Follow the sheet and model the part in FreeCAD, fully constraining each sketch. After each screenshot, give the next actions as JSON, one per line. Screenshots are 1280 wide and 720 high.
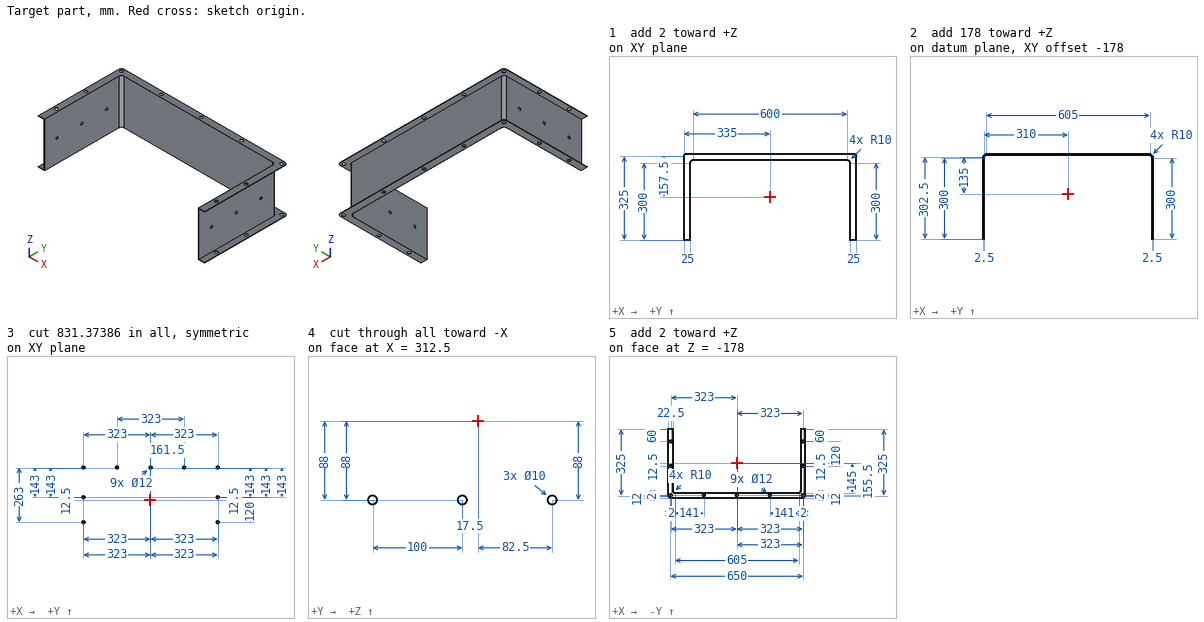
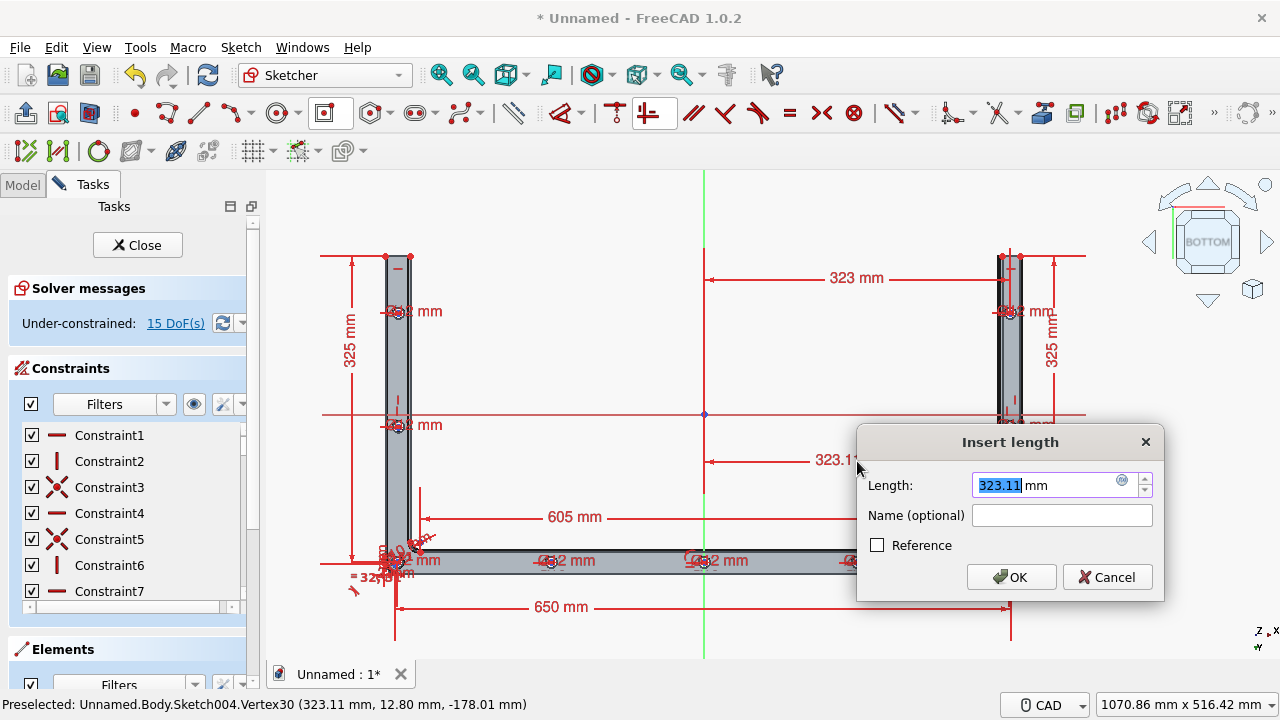
{"action": "type", "text": "323"}
{"action": "key", "text": "Return"}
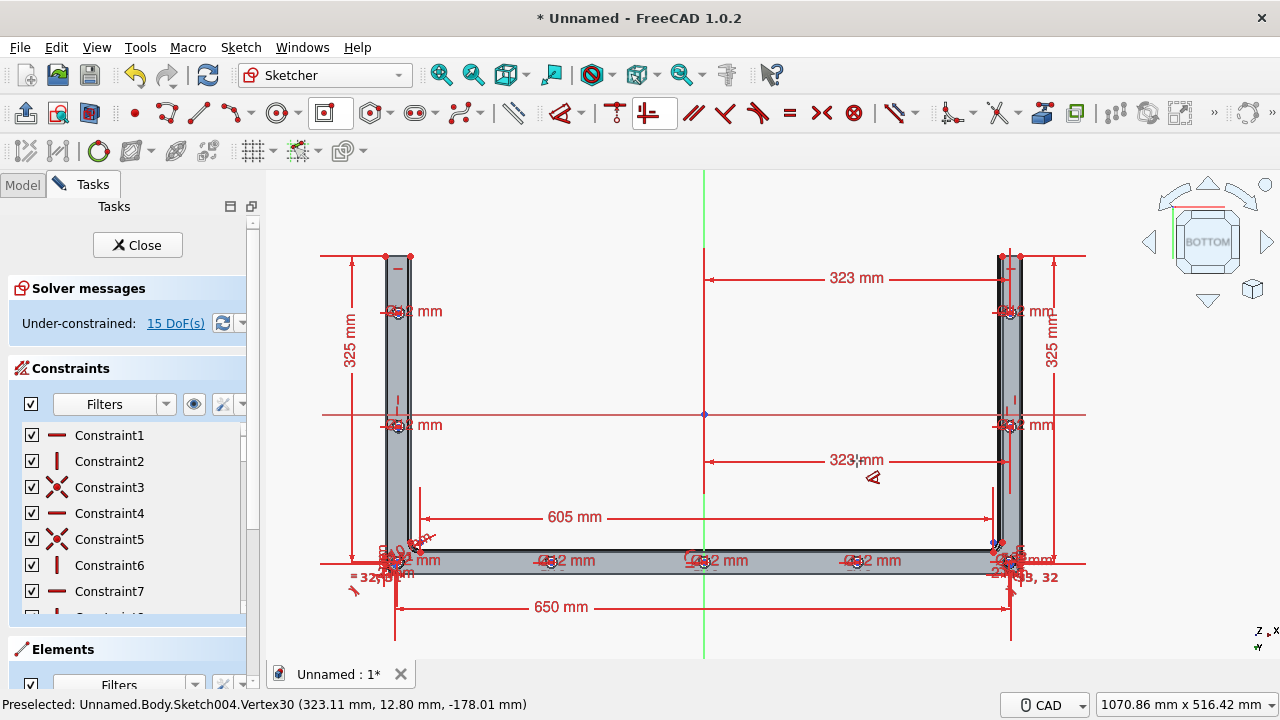
{"action": "left_click", "coordinate": [399, 313]}
{"action": "left_click", "coordinate": [551, 279]}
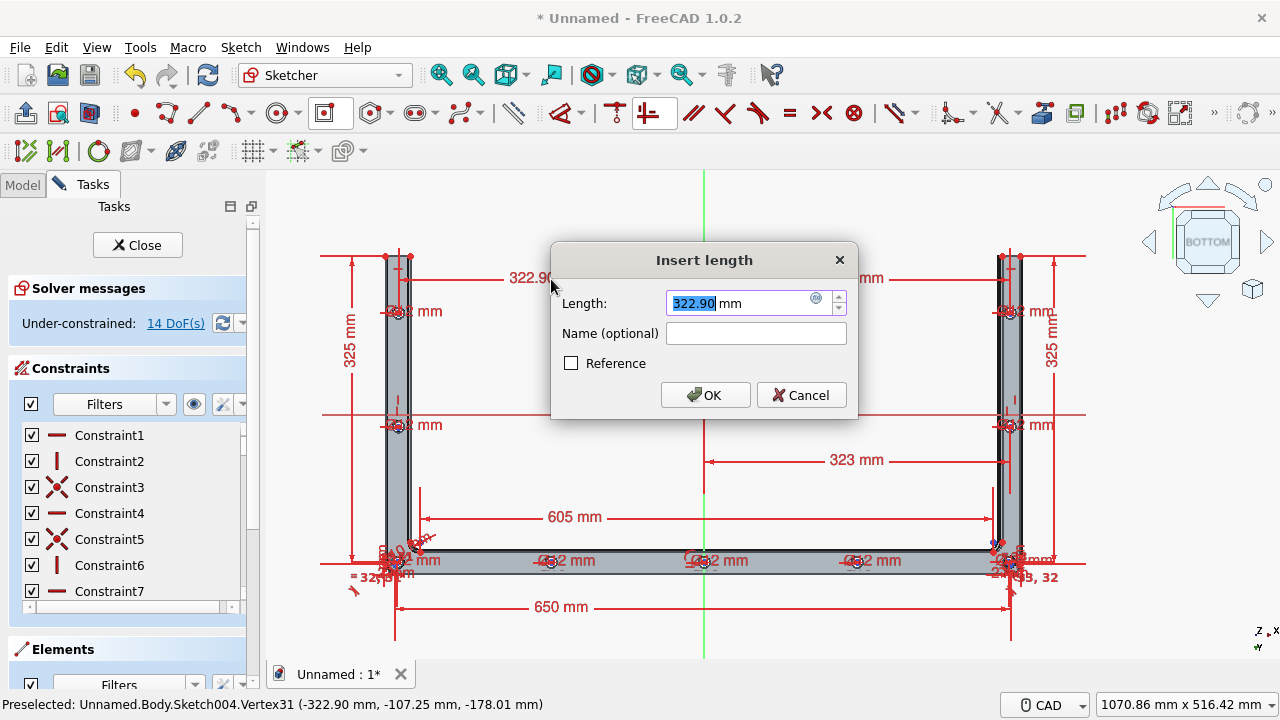
{"action": "type", "text": "323"}
{"action": "key", "text": "Return"}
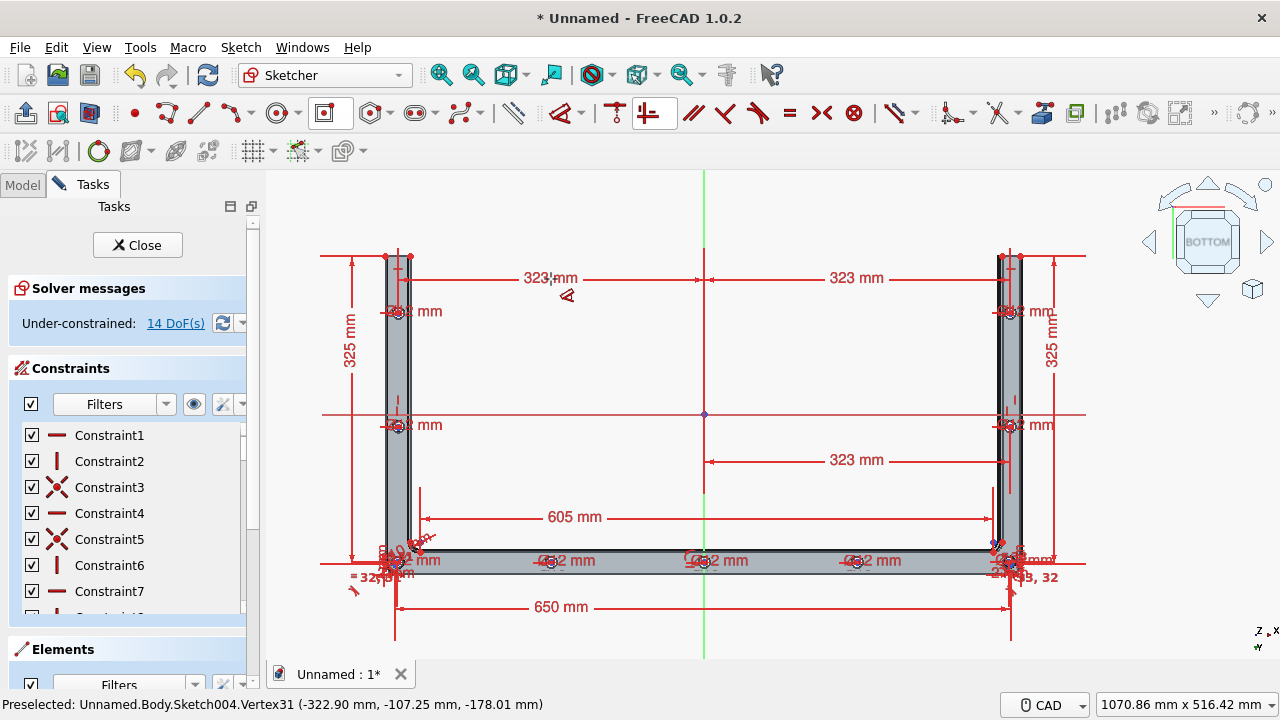
{"action": "left_click", "coordinate": [399, 427]}
{"action": "left_click", "coordinate": [551, 461]}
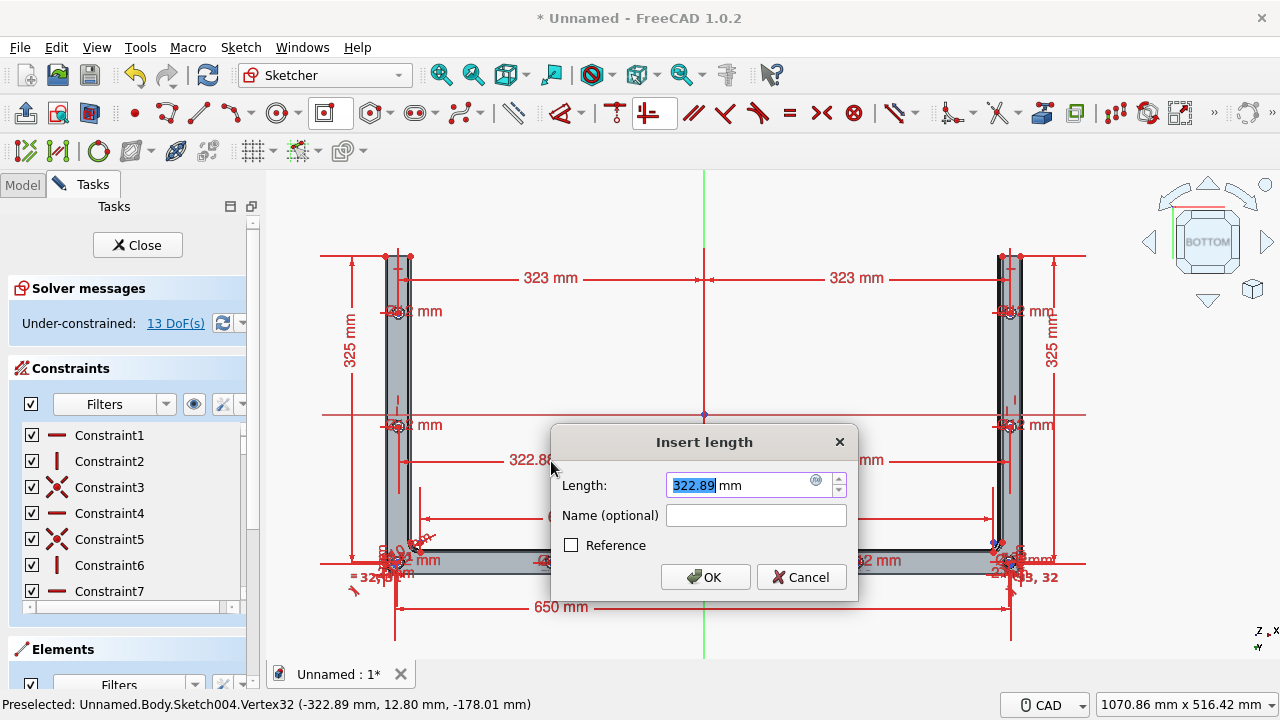
{"action": "type", "text": "323"}
{"action": "key", "text": "Return"}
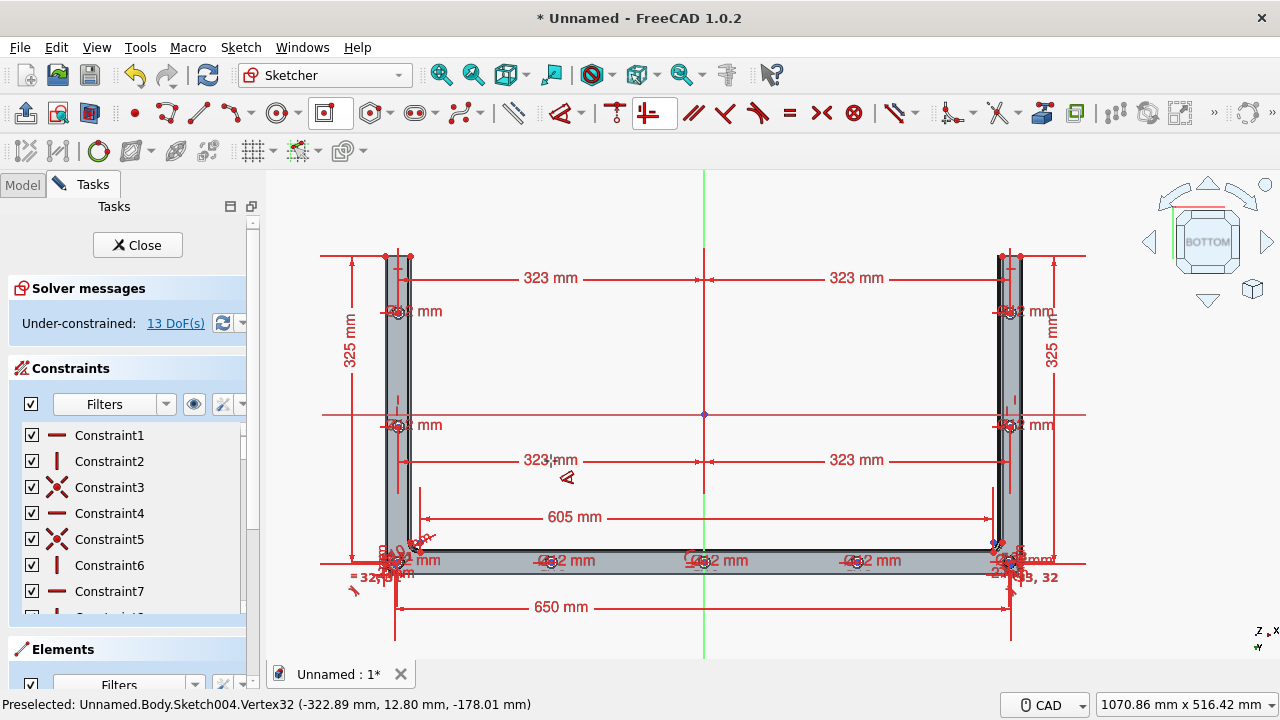
{"action": "scroll", "coordinate": [1009, 562], "scroll_direction": "up", "scroll_amount": 8}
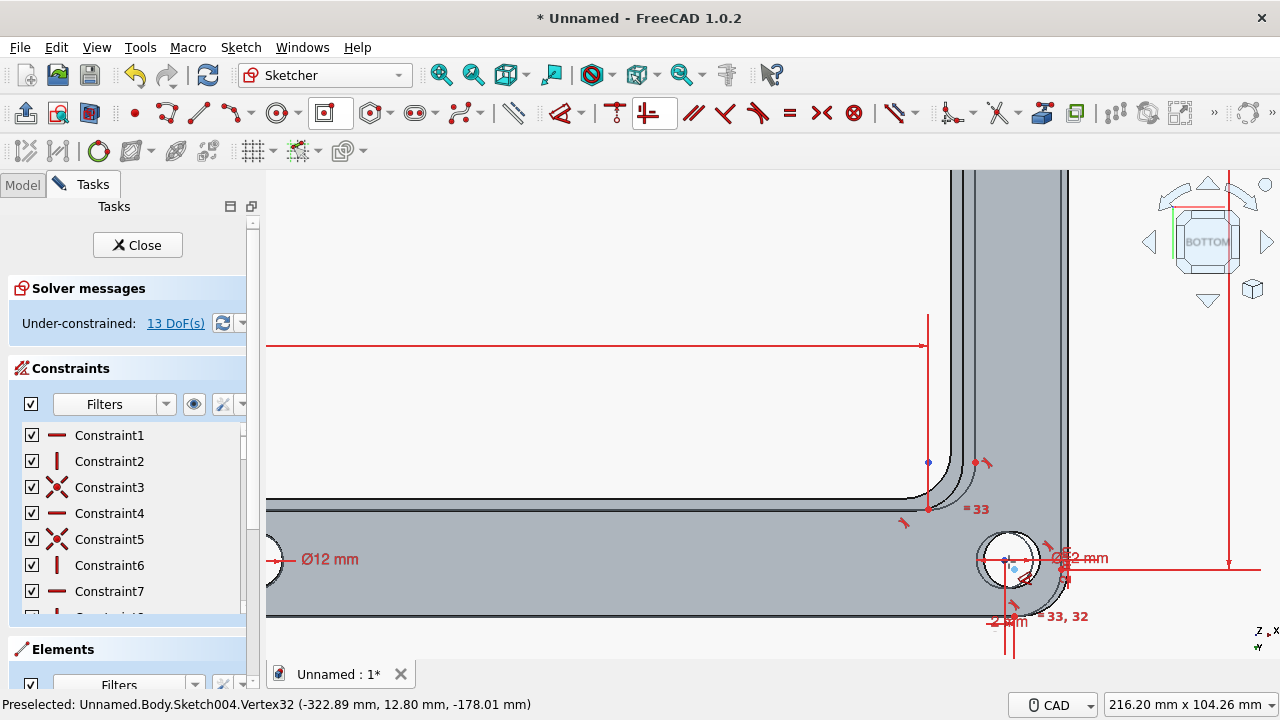
{"action": "left_click", "coordinate": [1005, 560]}
{"action": "left_click", "coordinate": [649, 594]}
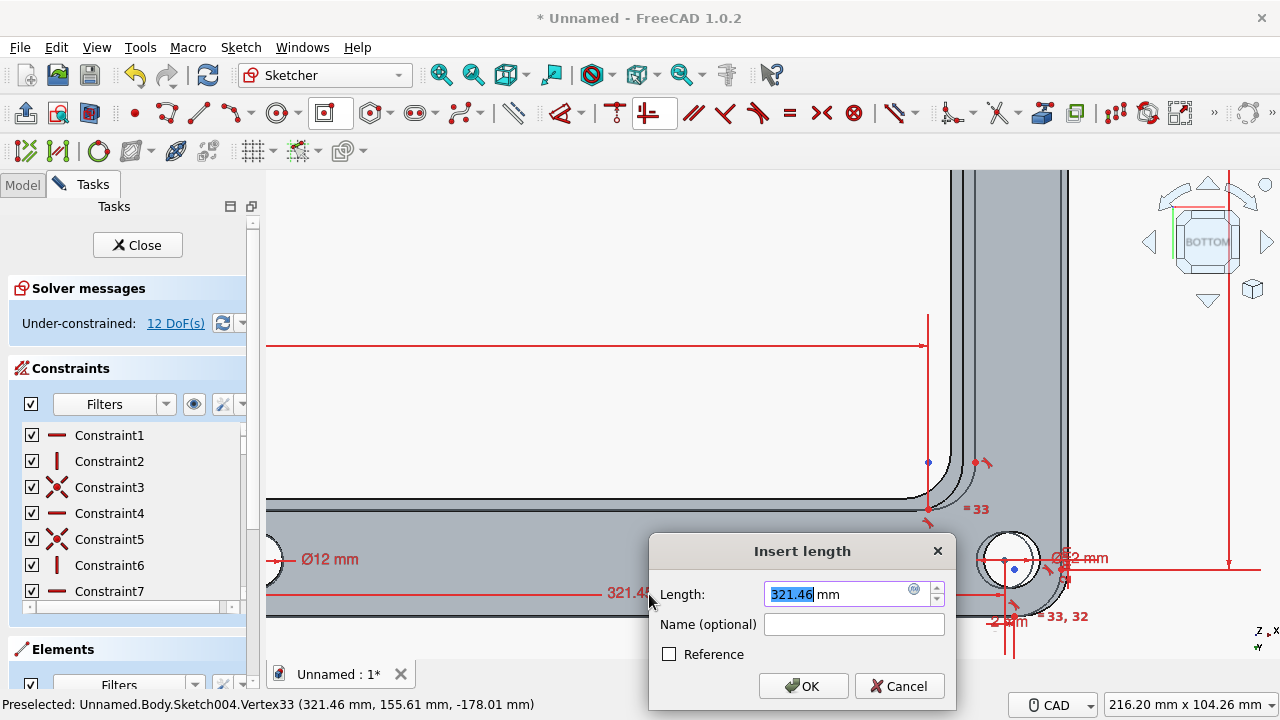
{"action": "type", "text": "323"}
{"action": "key", "text": "Return"}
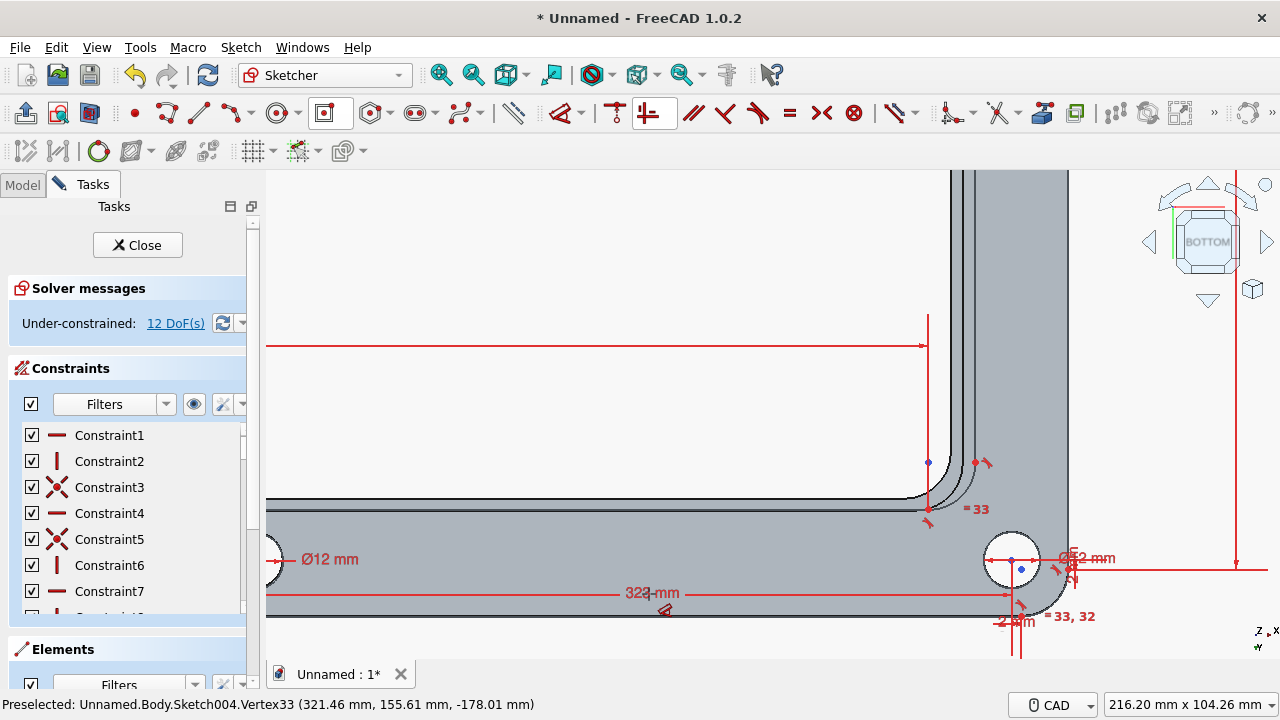
{"action": "scroll", "coordinate": [1010, 562], "scroll_direction": "down", "scroll_amount": 8}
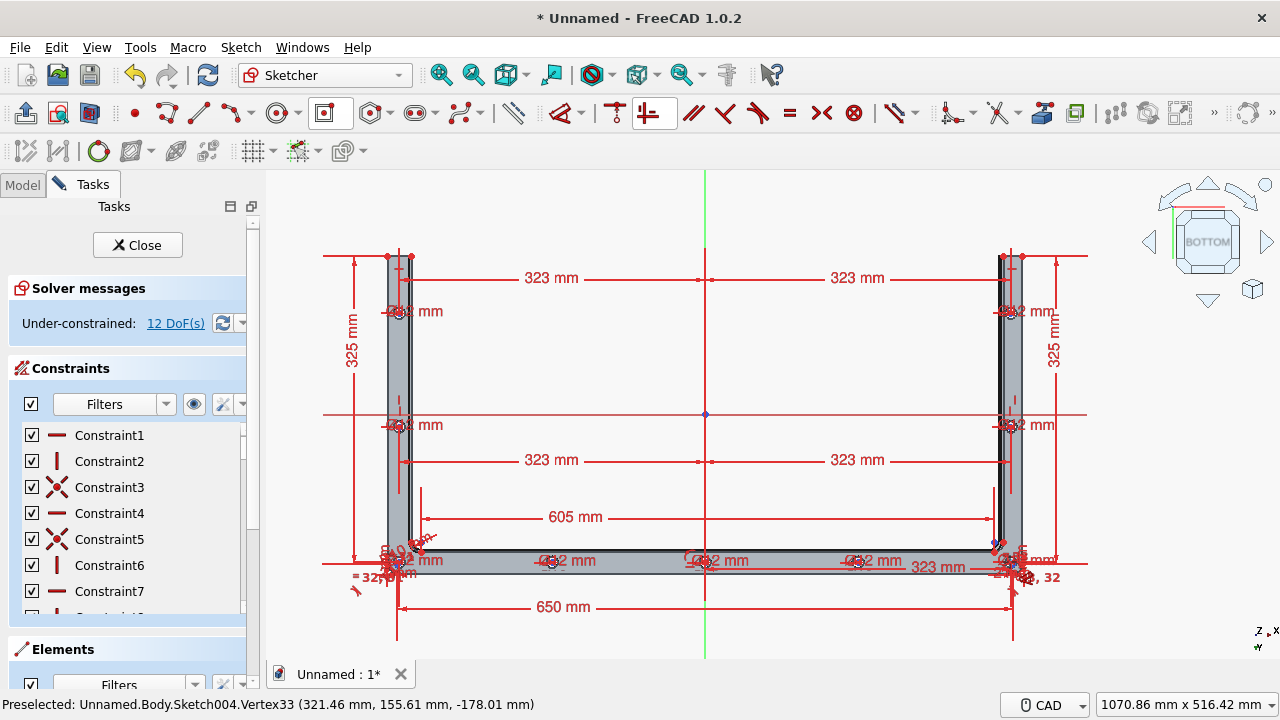
{"action": "left_click", "coordinate": [1004, 256]}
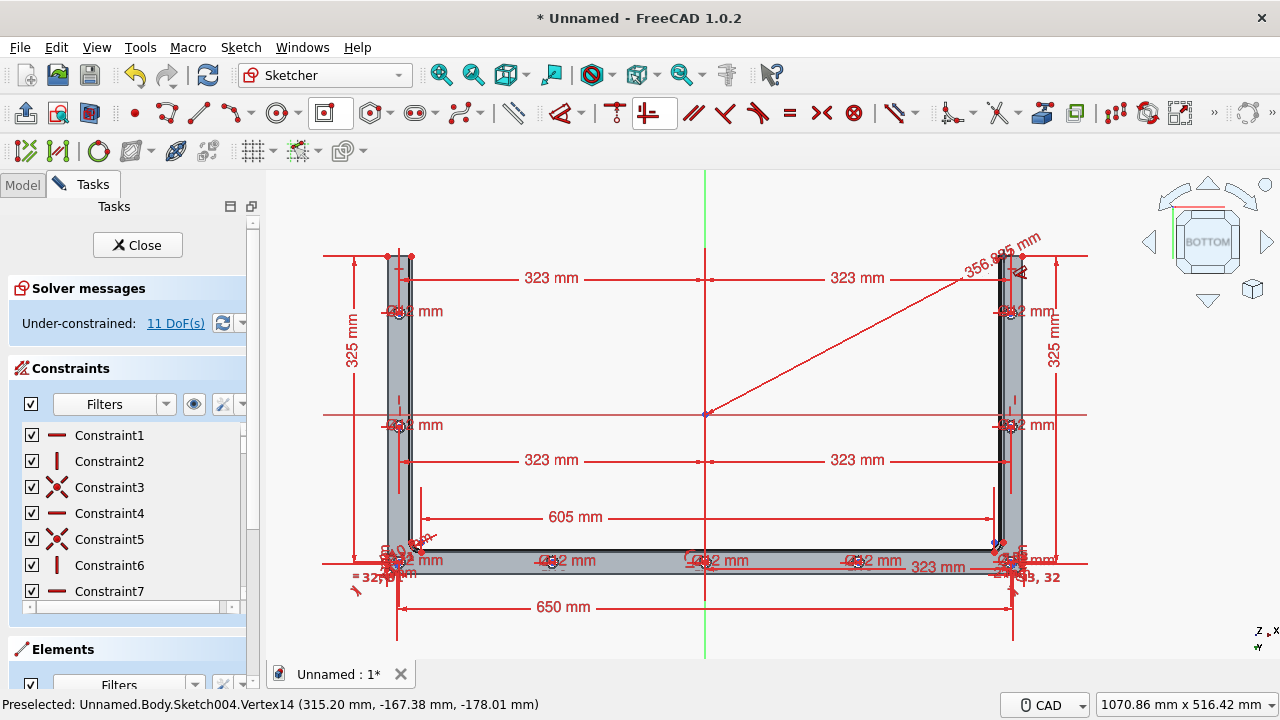
{"action": "left_click", "coordinate": [1011, 313]}
{"action": "left_click", "coordinate": [1045, 285]}